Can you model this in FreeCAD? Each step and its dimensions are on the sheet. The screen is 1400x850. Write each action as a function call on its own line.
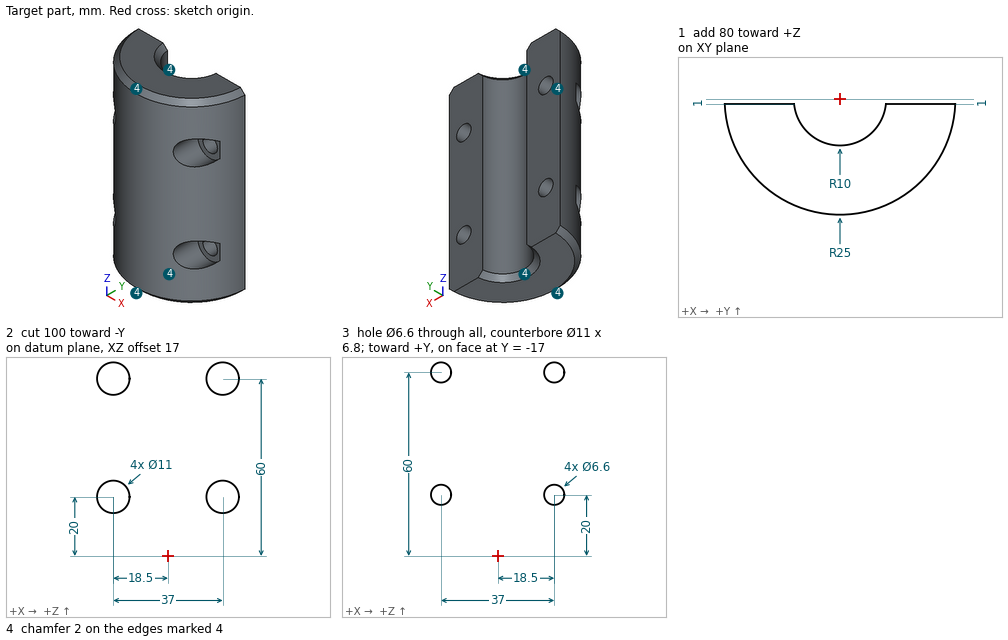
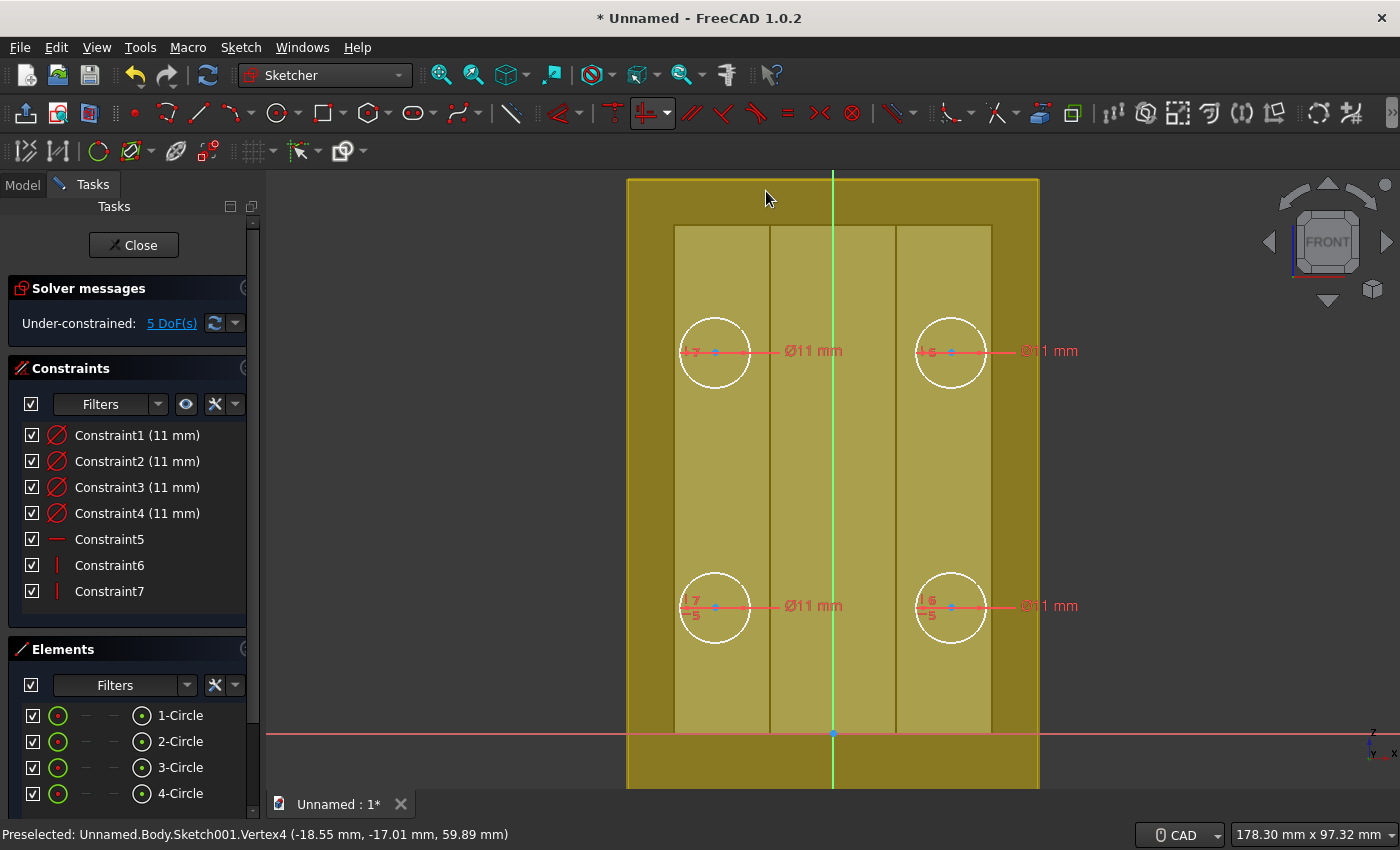
click(951, 353)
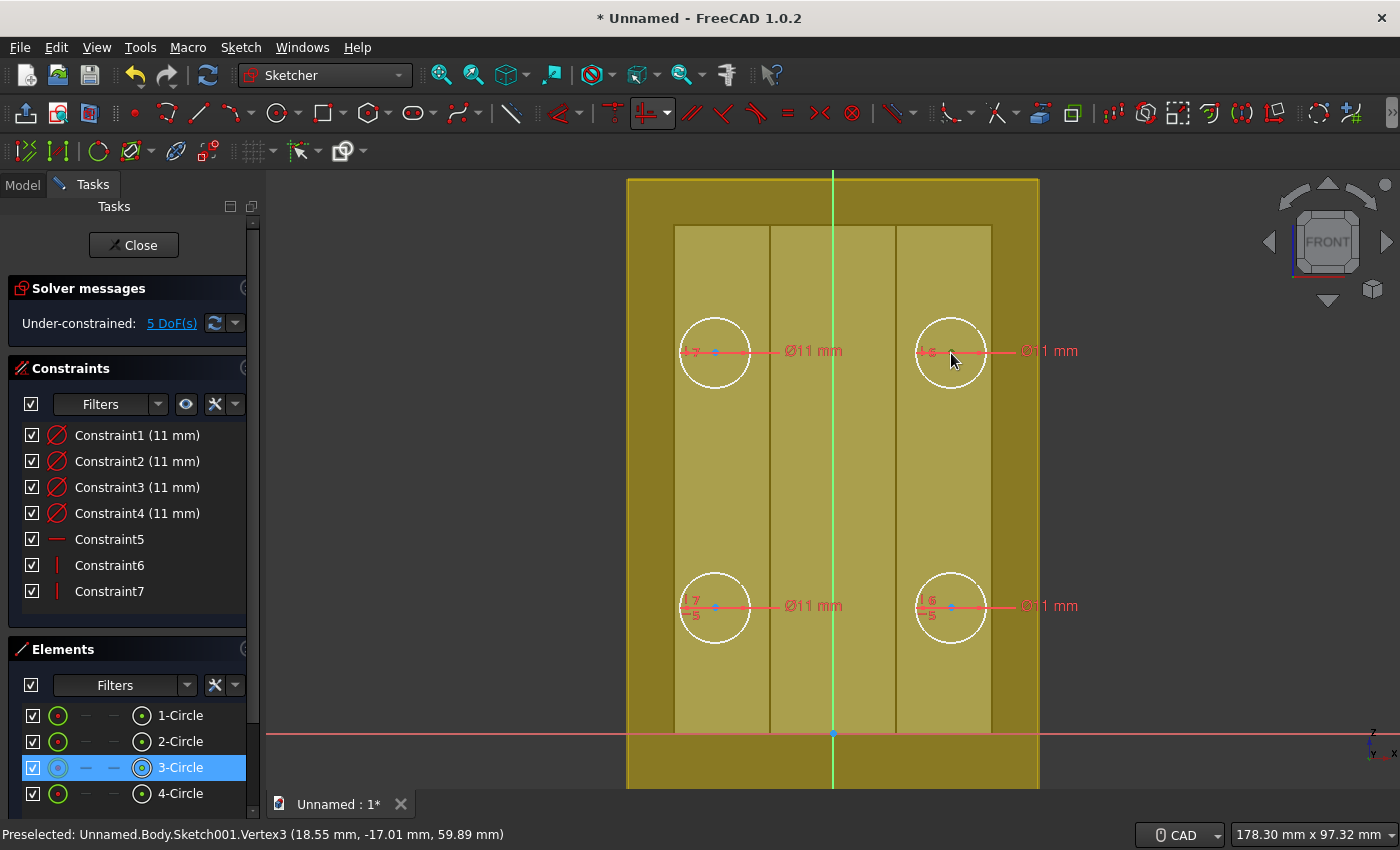
click(715, 353)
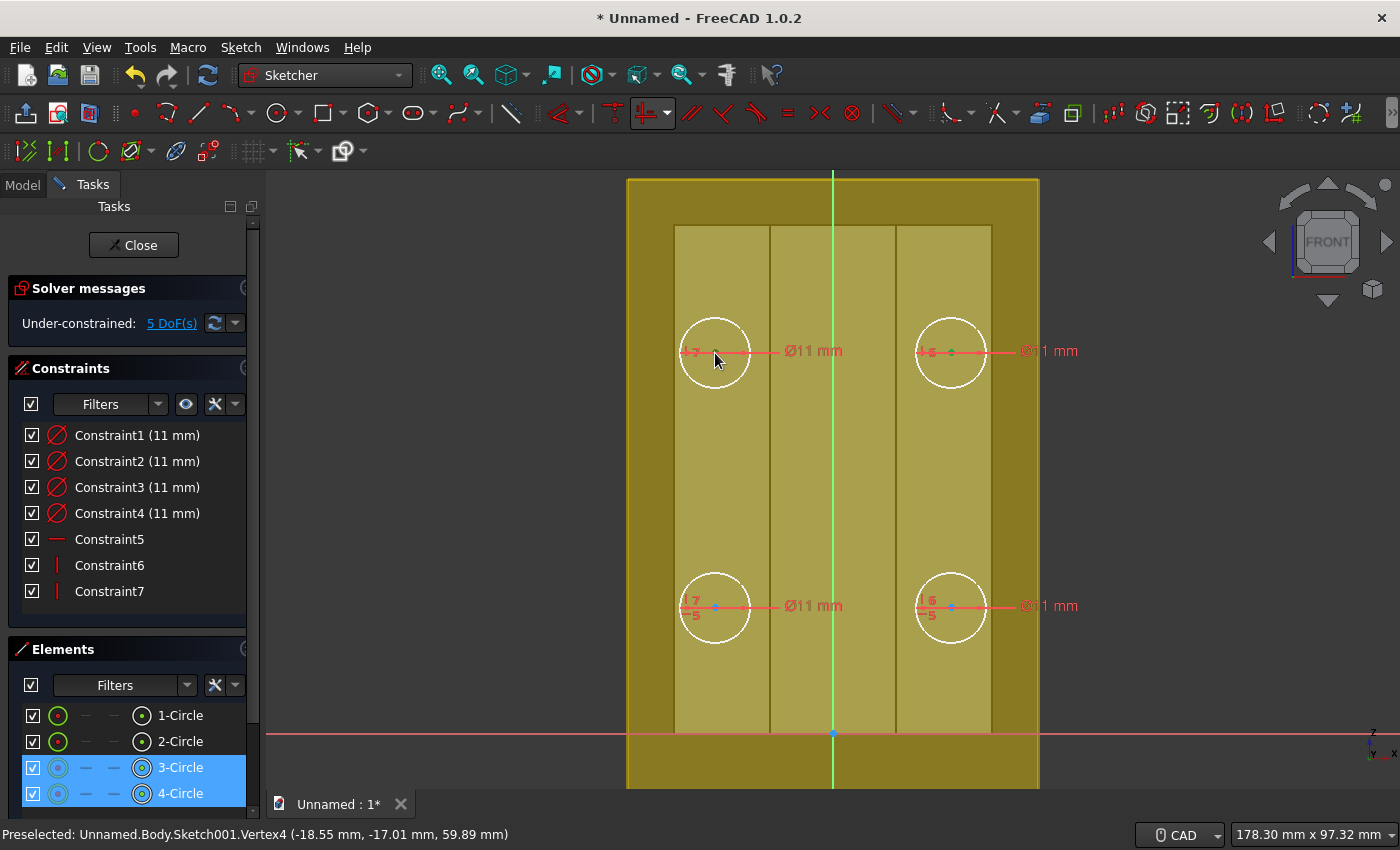
key(h)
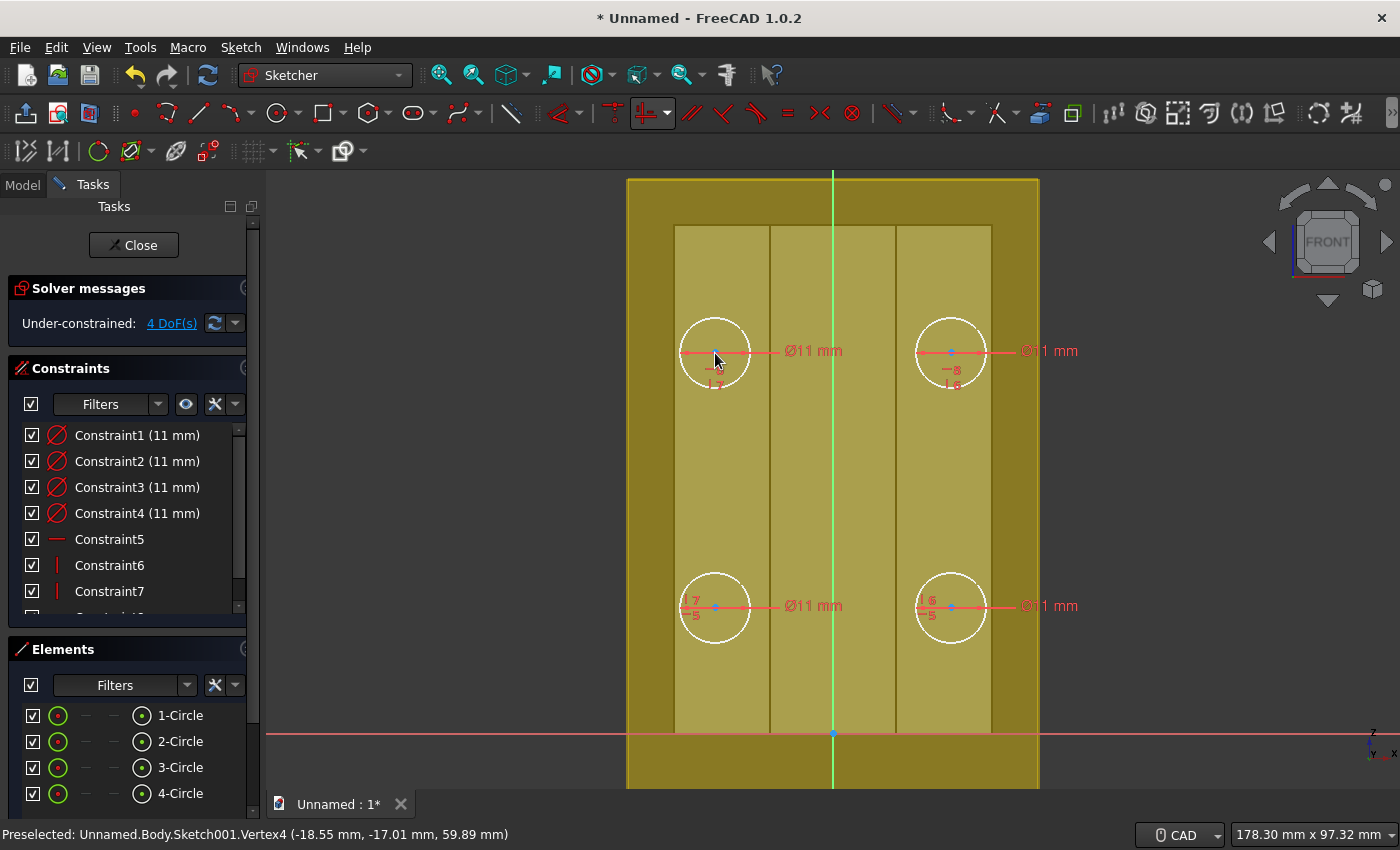
click(558, 114)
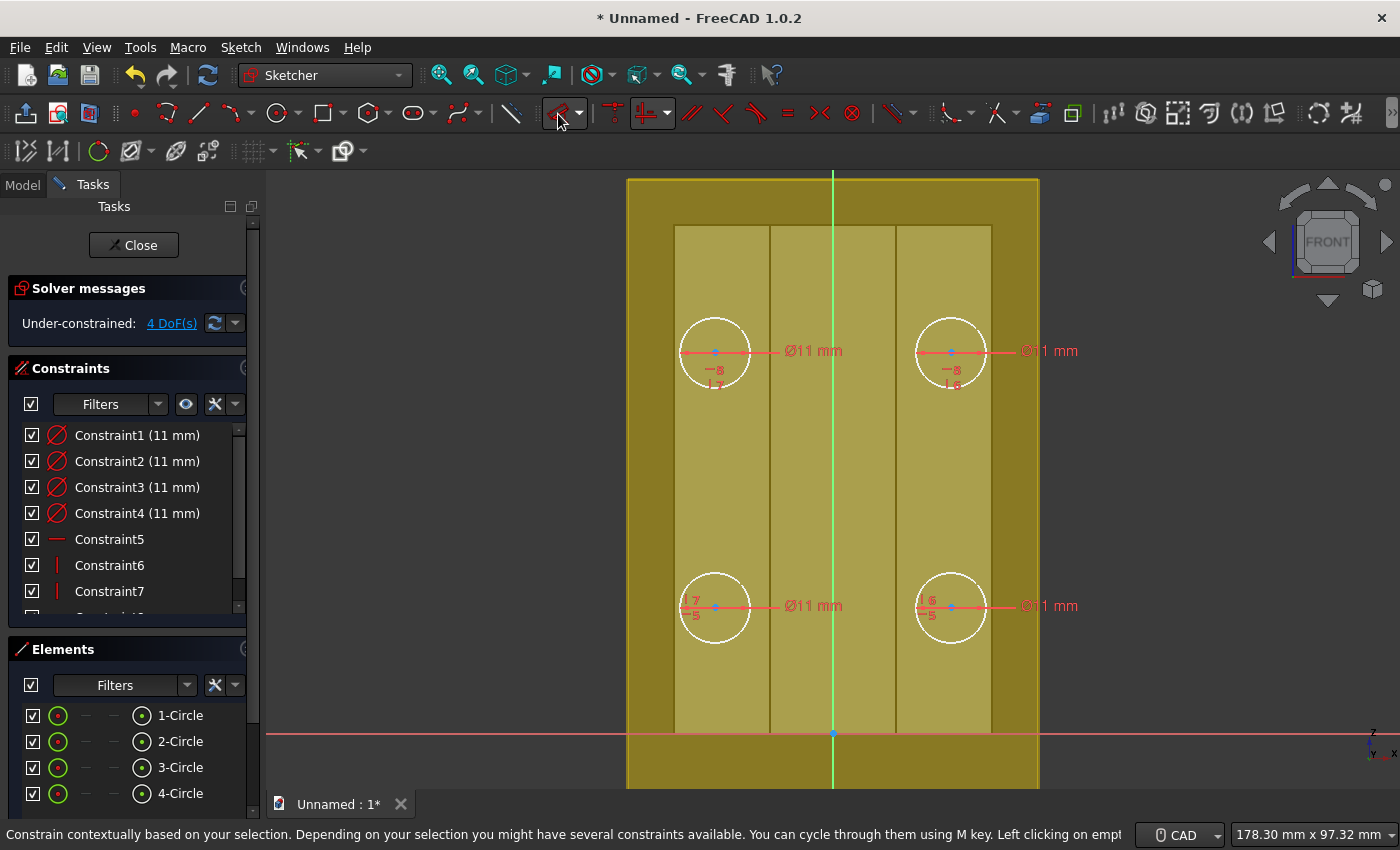
click(715, 608)
click(681, 671)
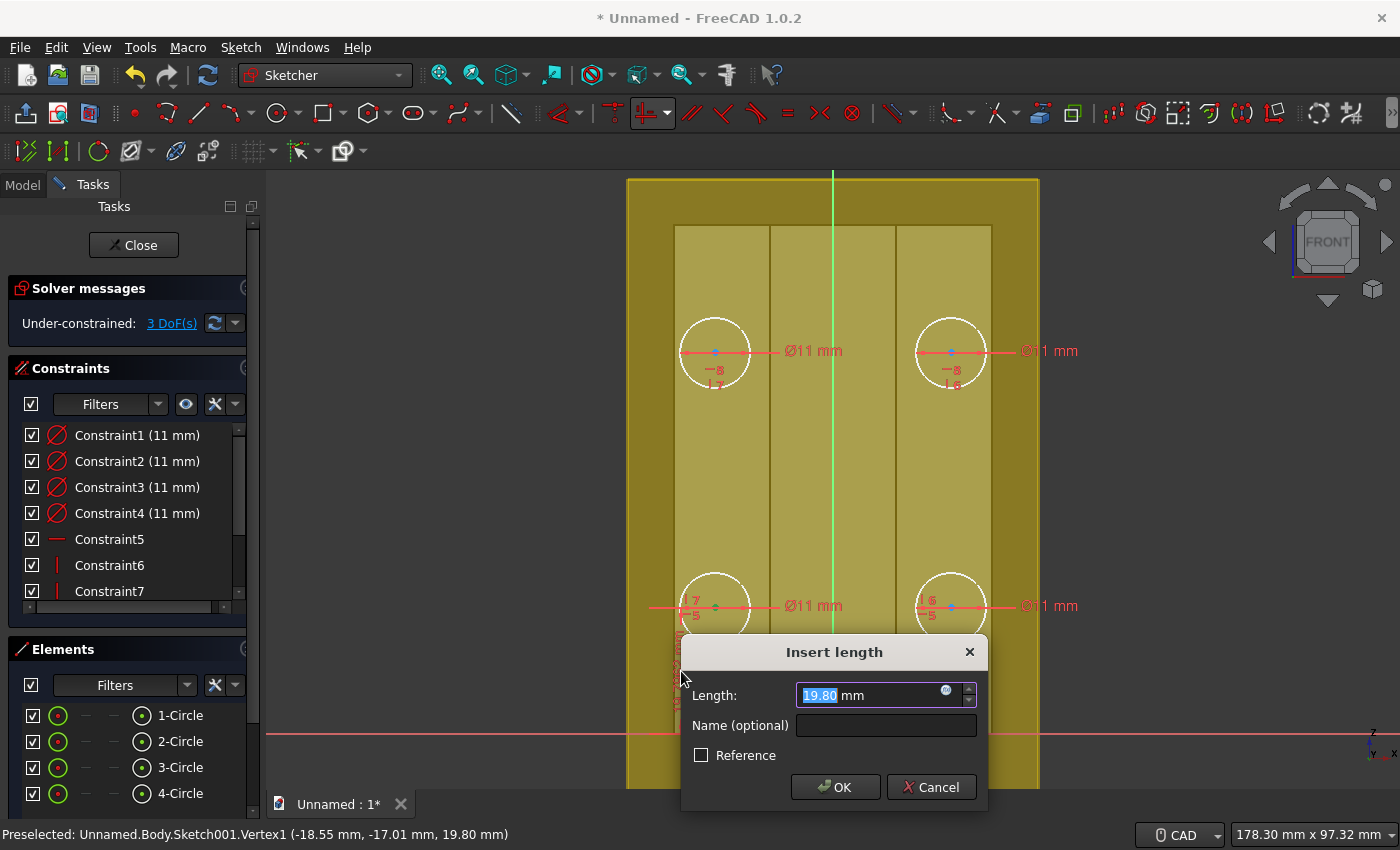
text(20)
key(Return)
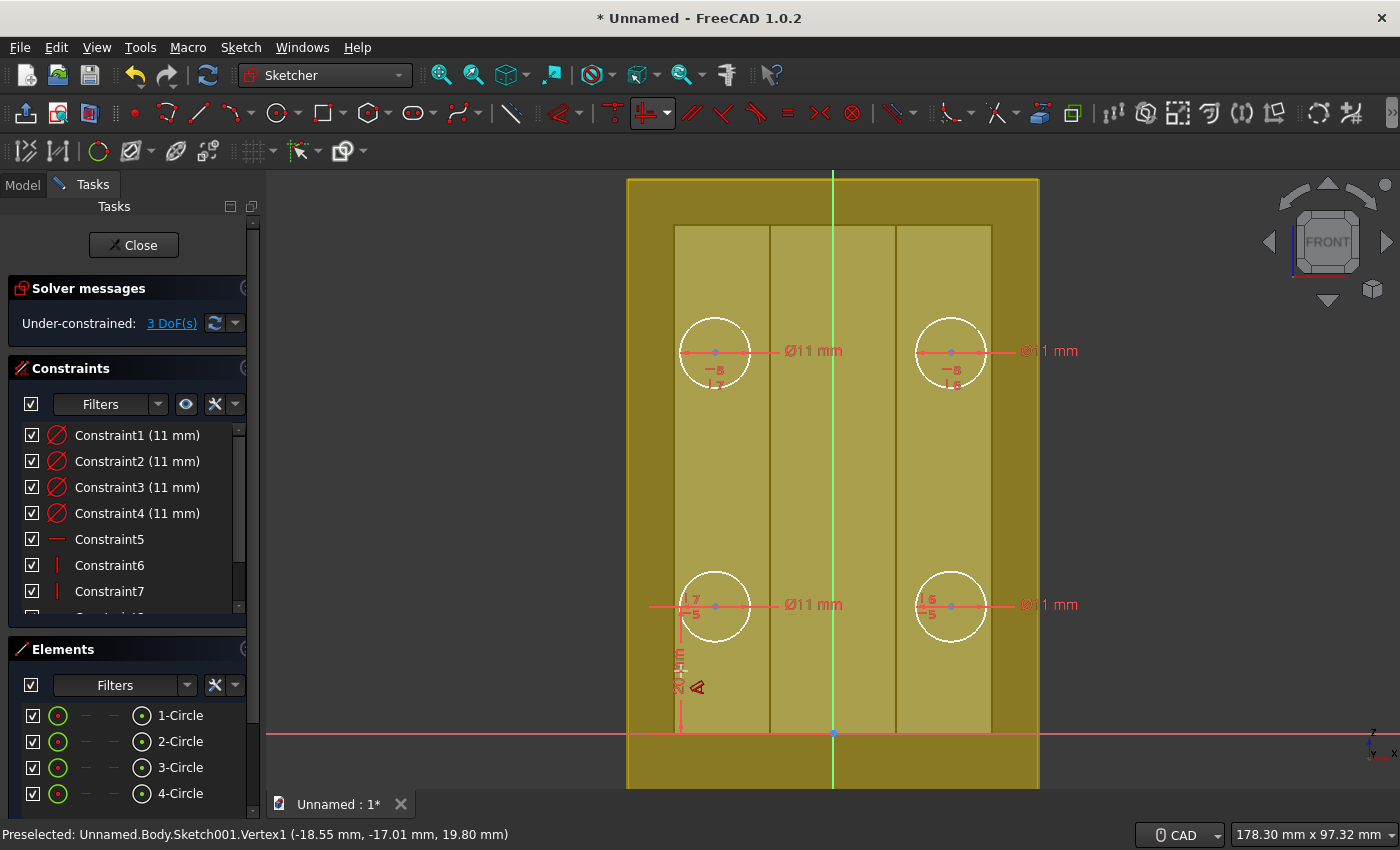
click(951, 353)
click(985, 543)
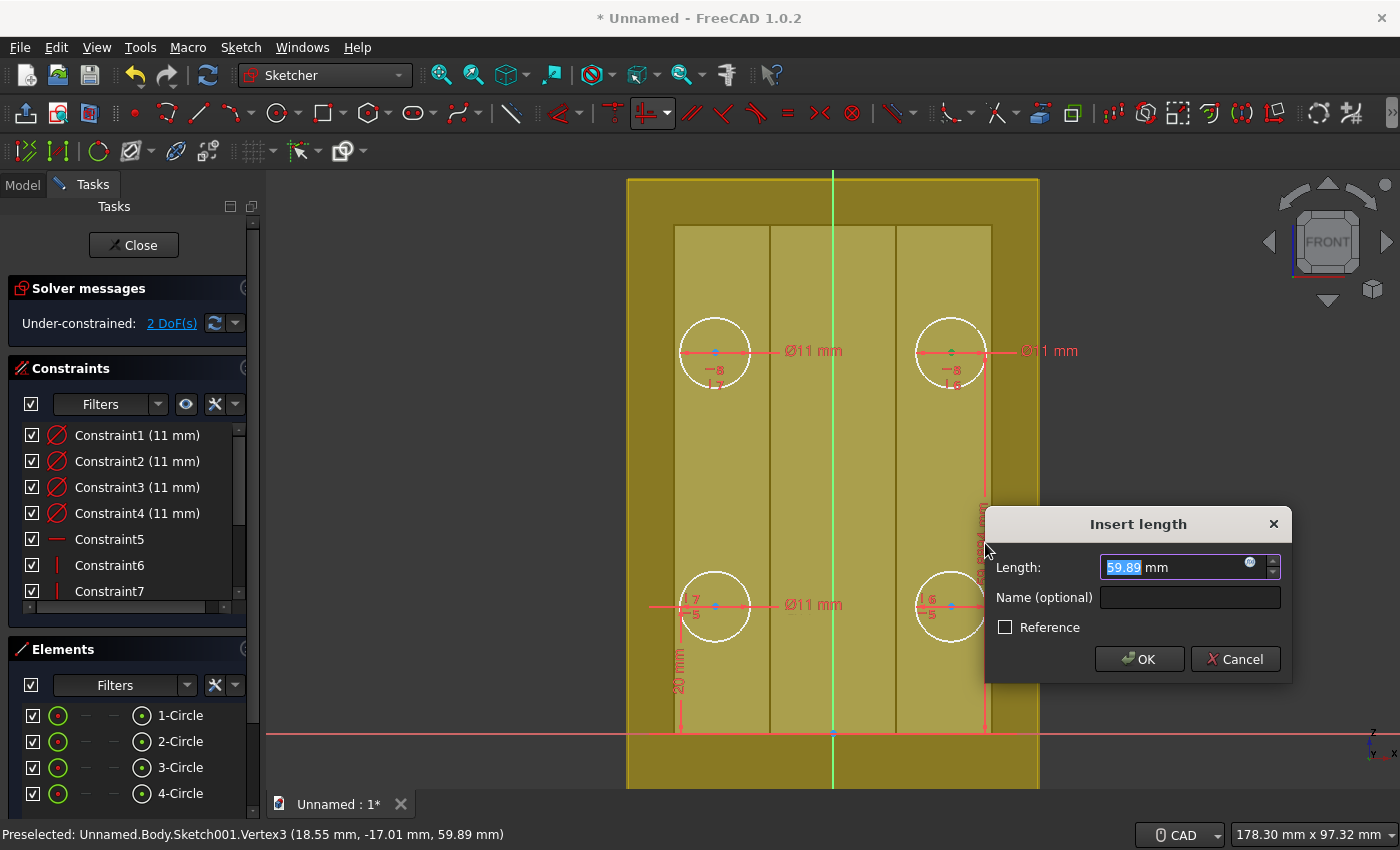
text(60)
key(Return)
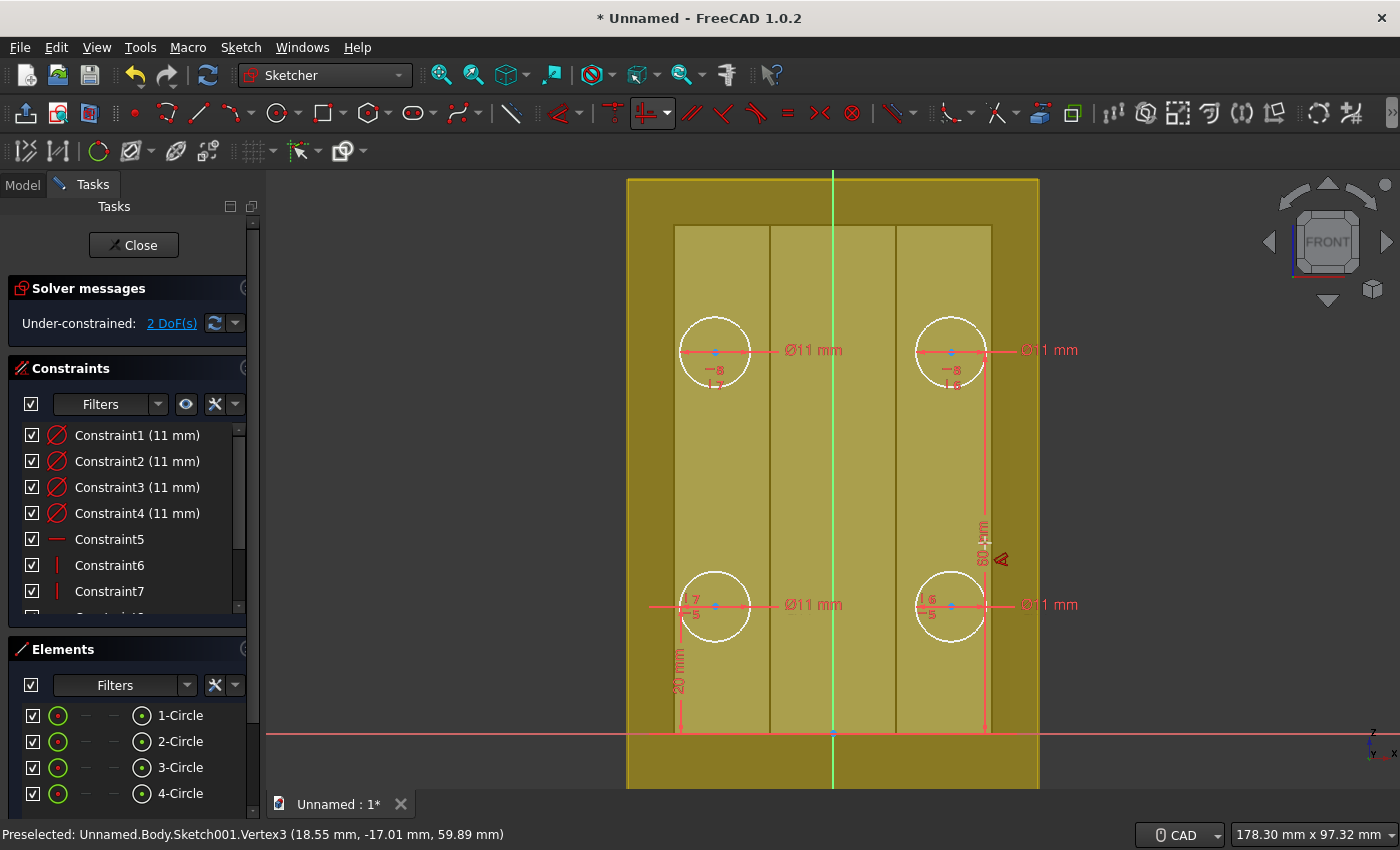
click(715, 607)